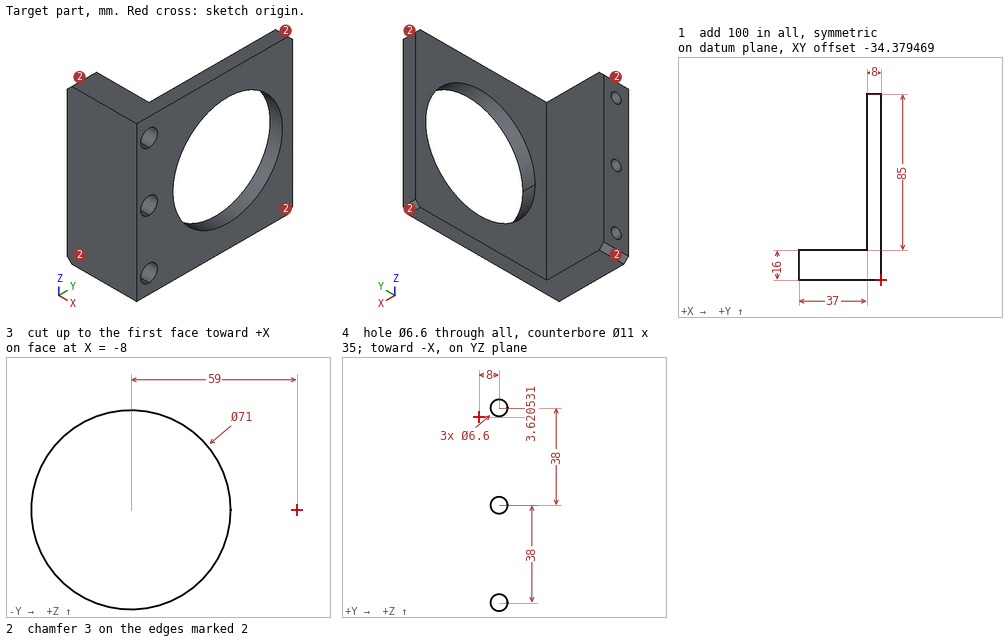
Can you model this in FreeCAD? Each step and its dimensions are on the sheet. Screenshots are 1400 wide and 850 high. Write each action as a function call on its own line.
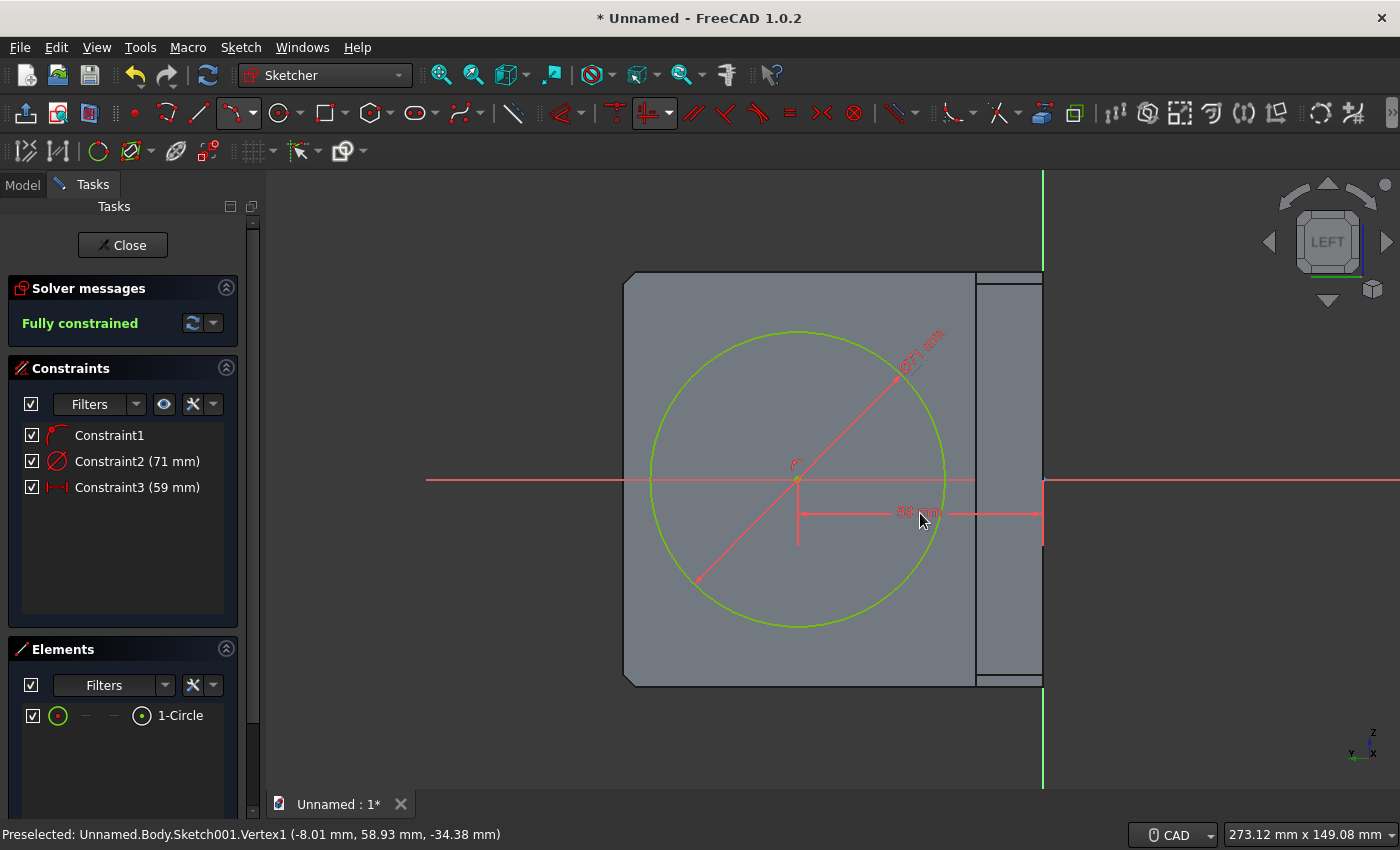
click(123, 245)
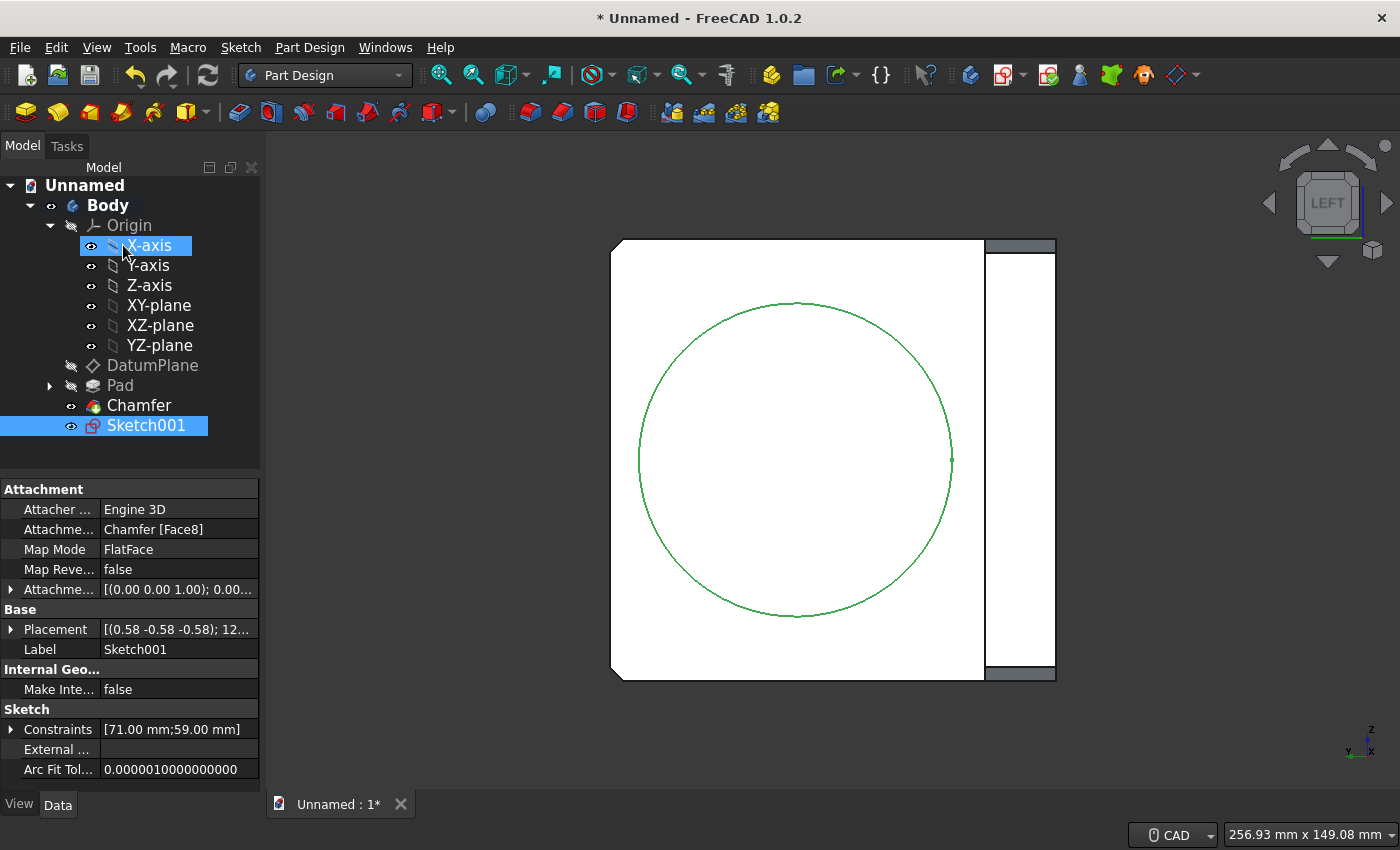
click(240, 112)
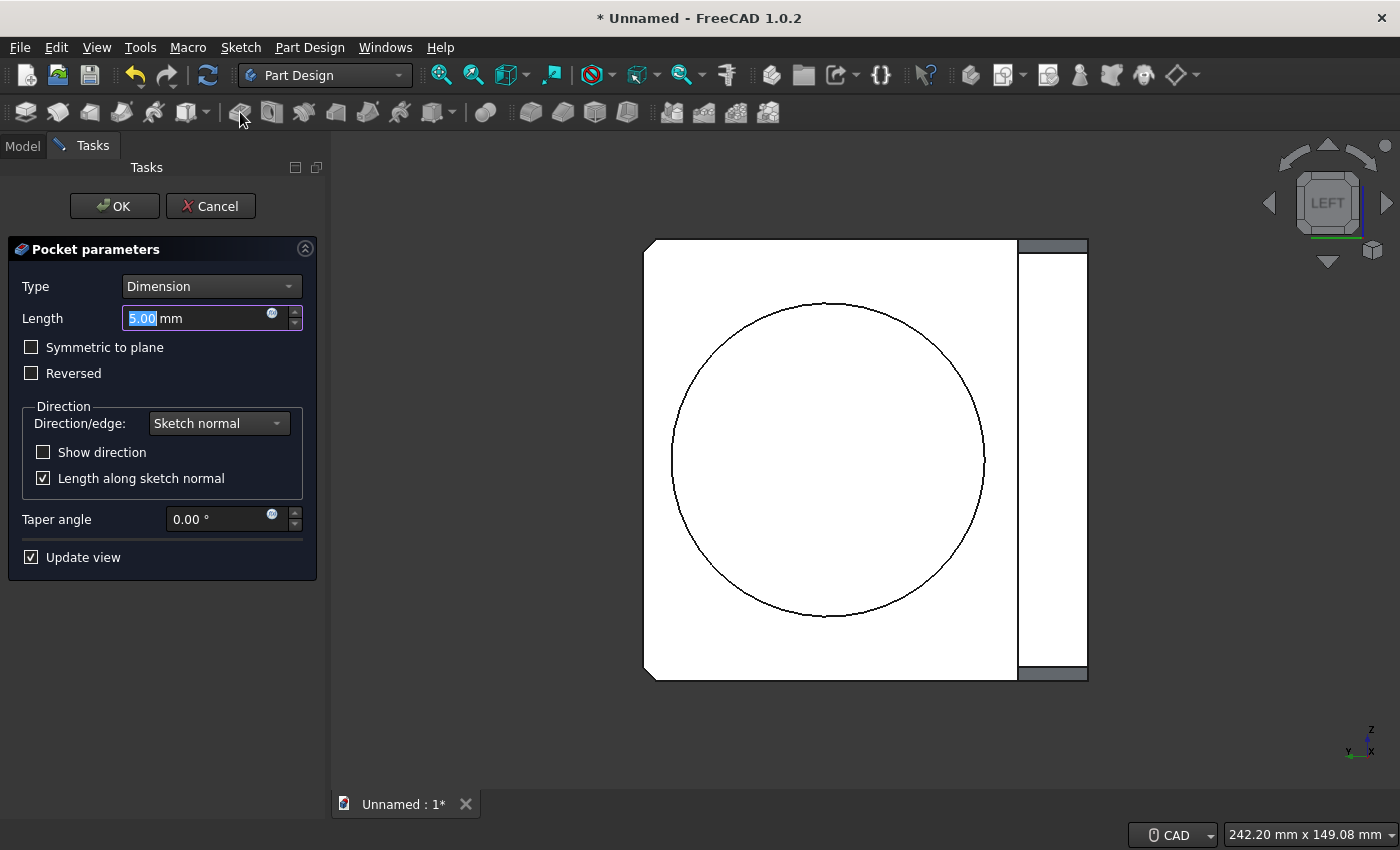
click(212, 286)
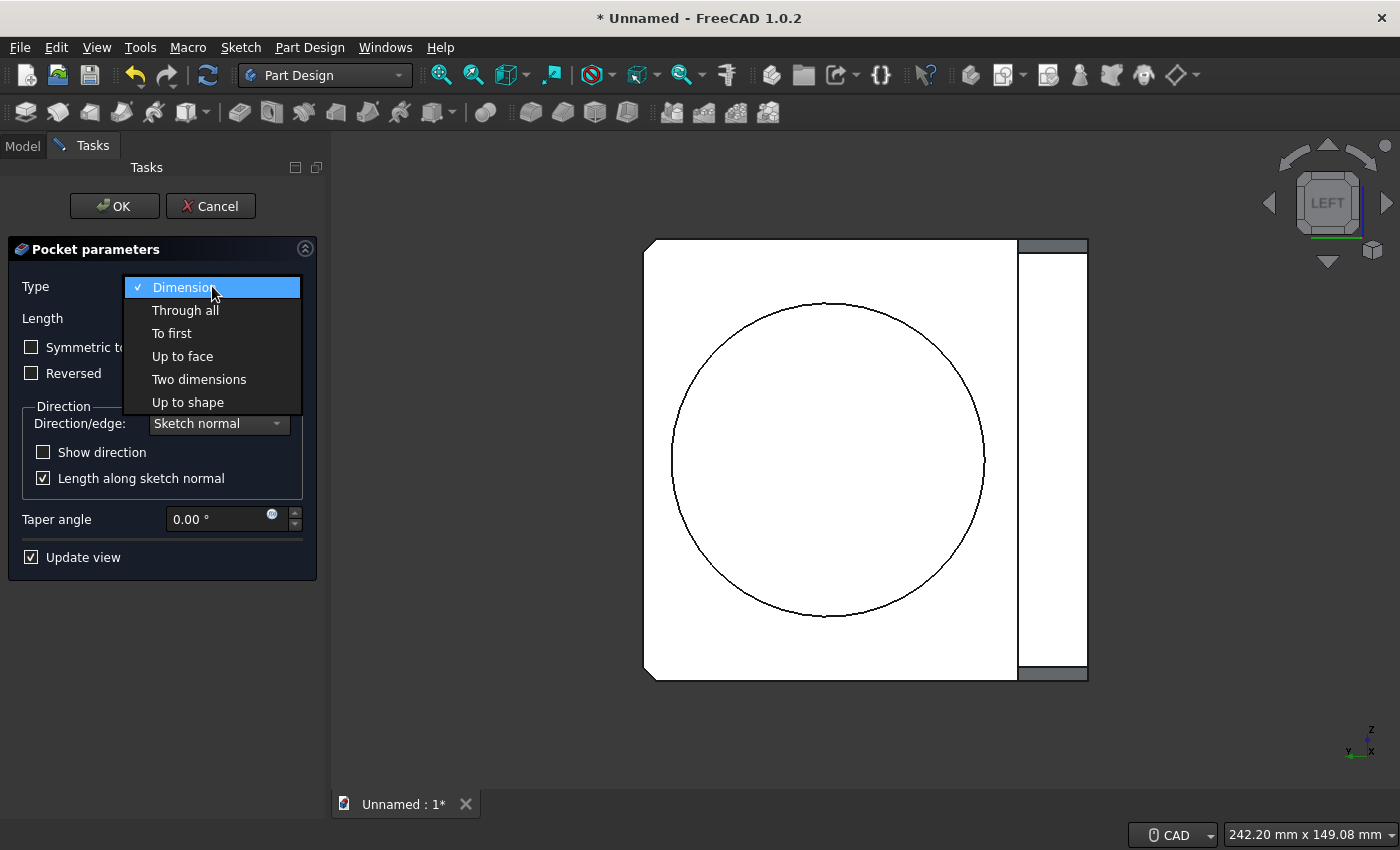
click(212, 334)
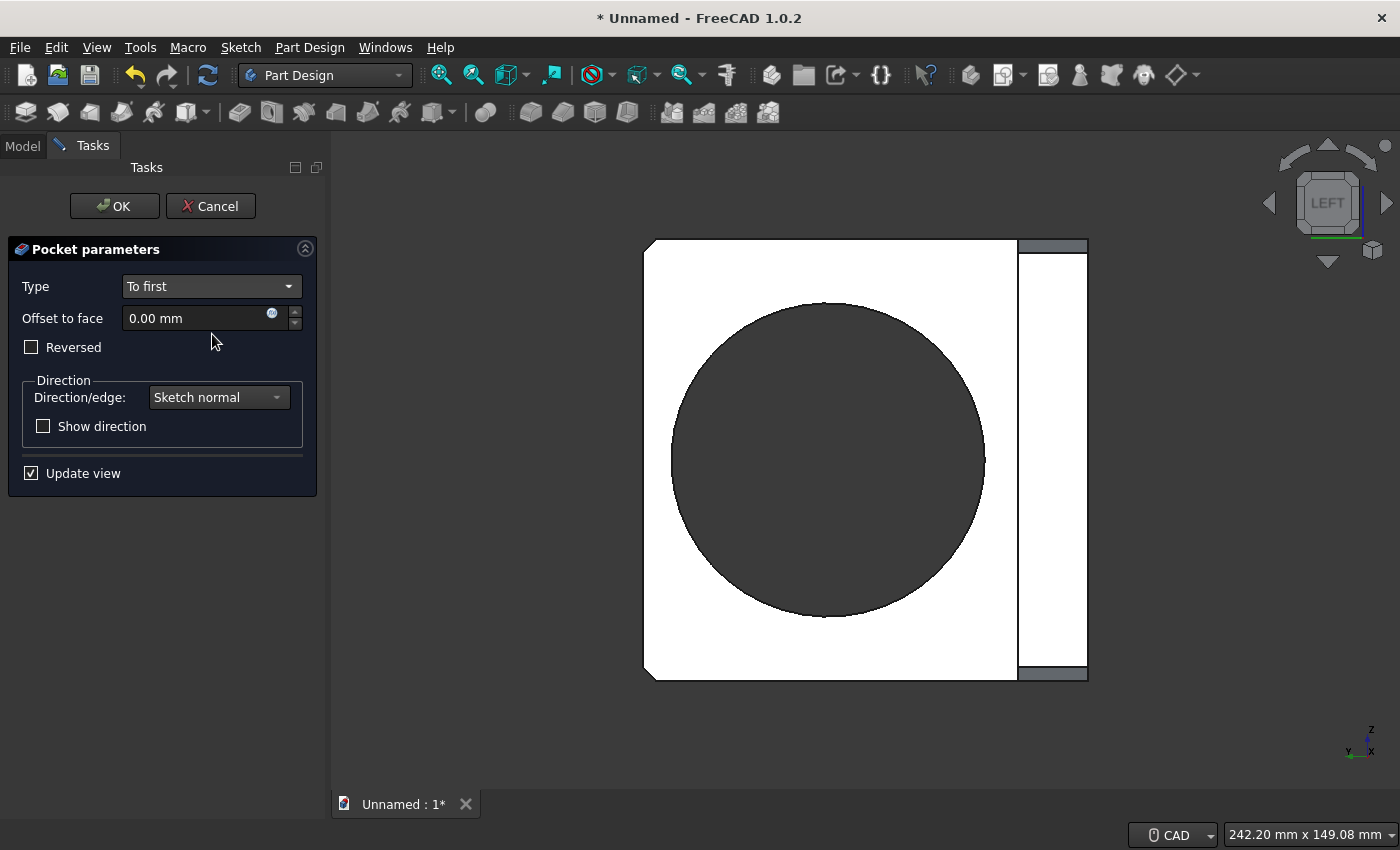
click(115, 206)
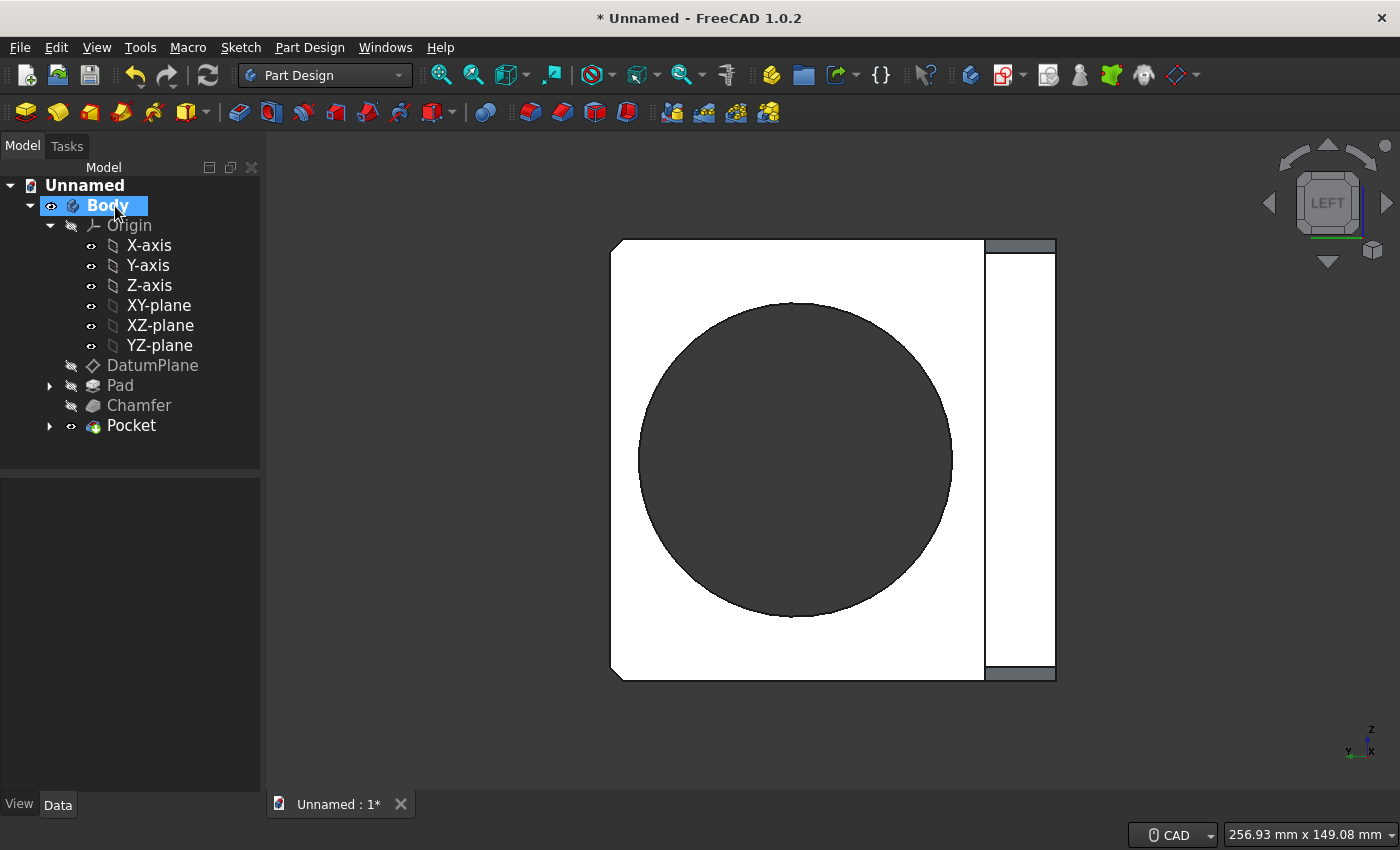
click(1004, 76)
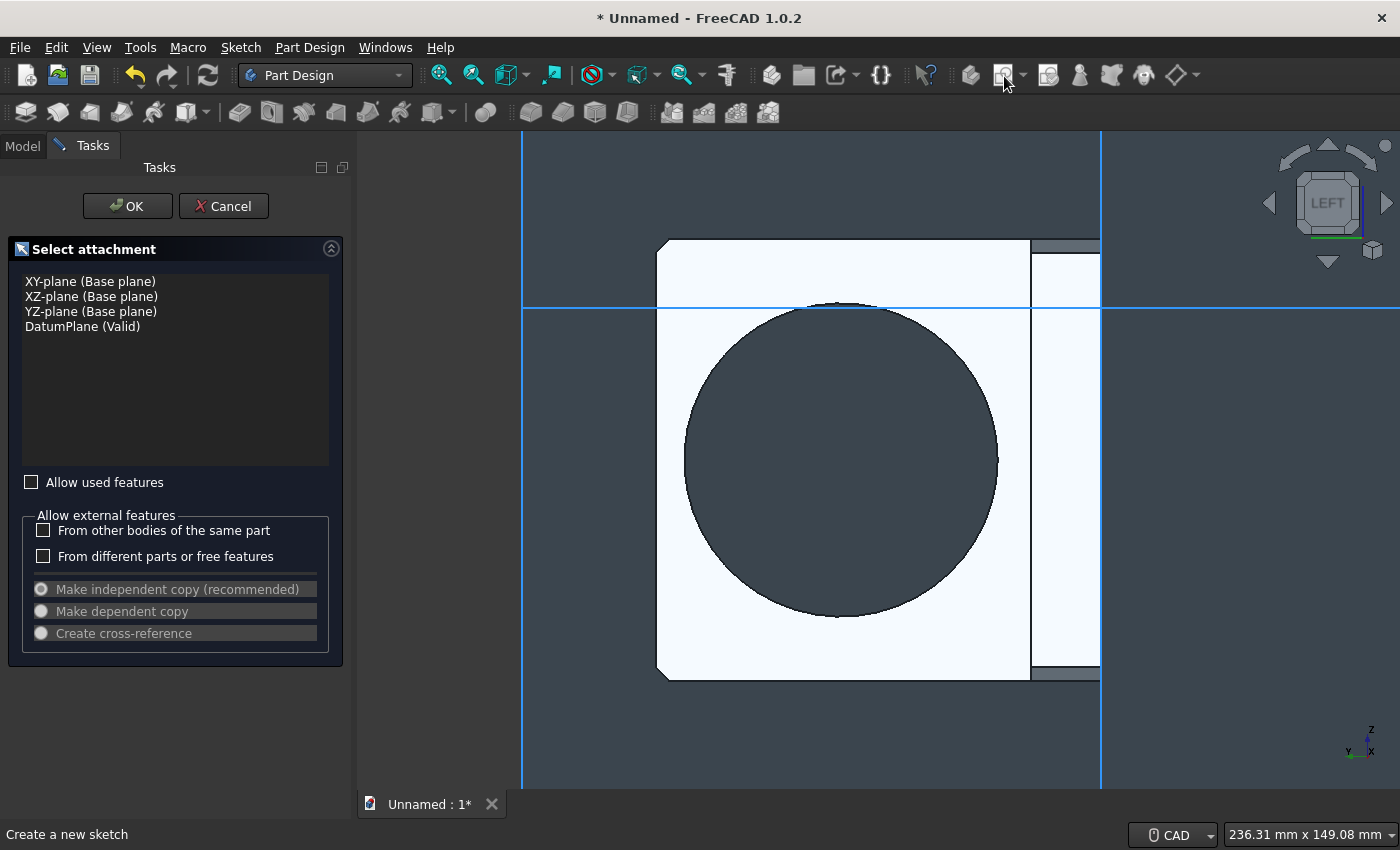
click(82, 312)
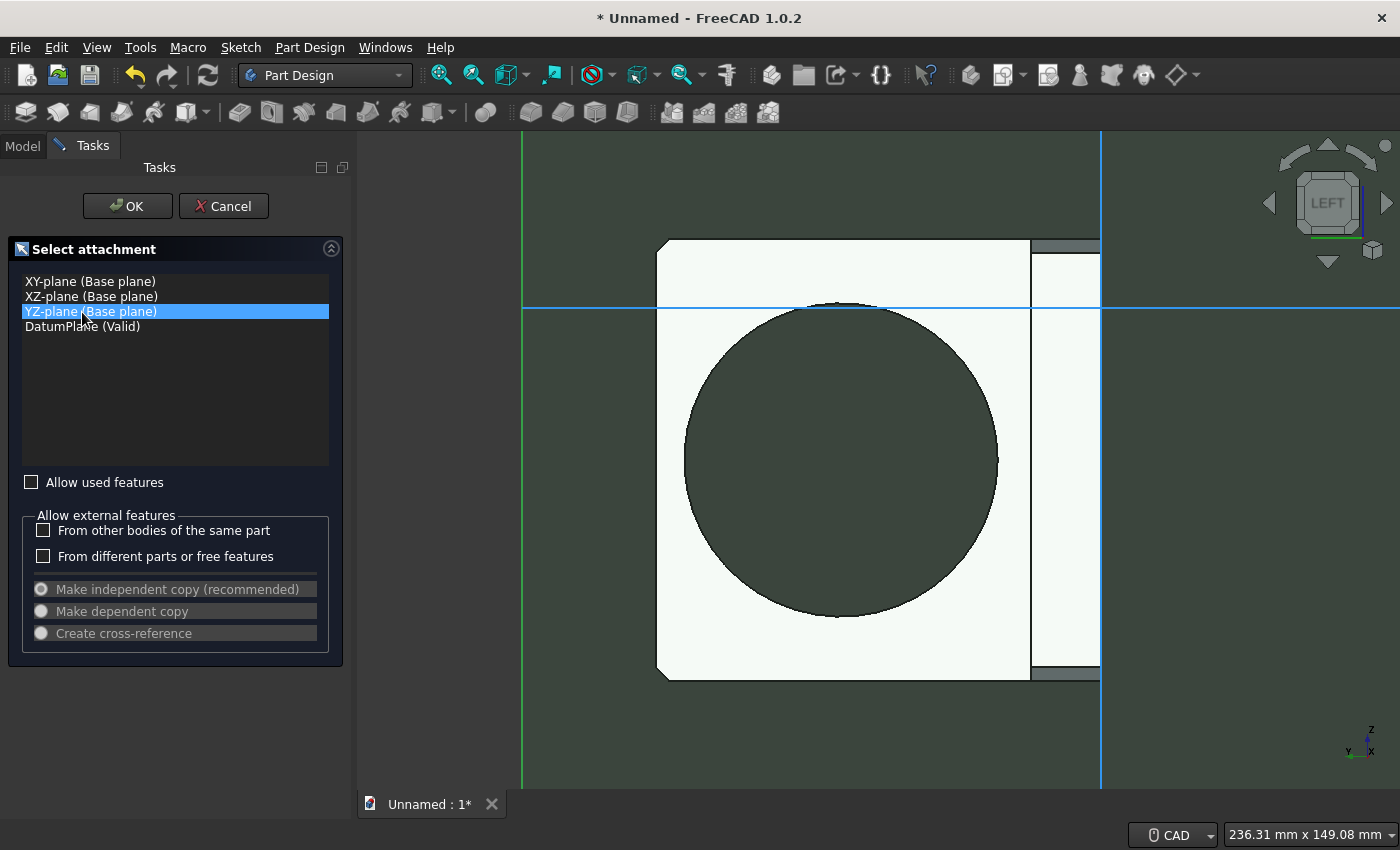
click(128, 206)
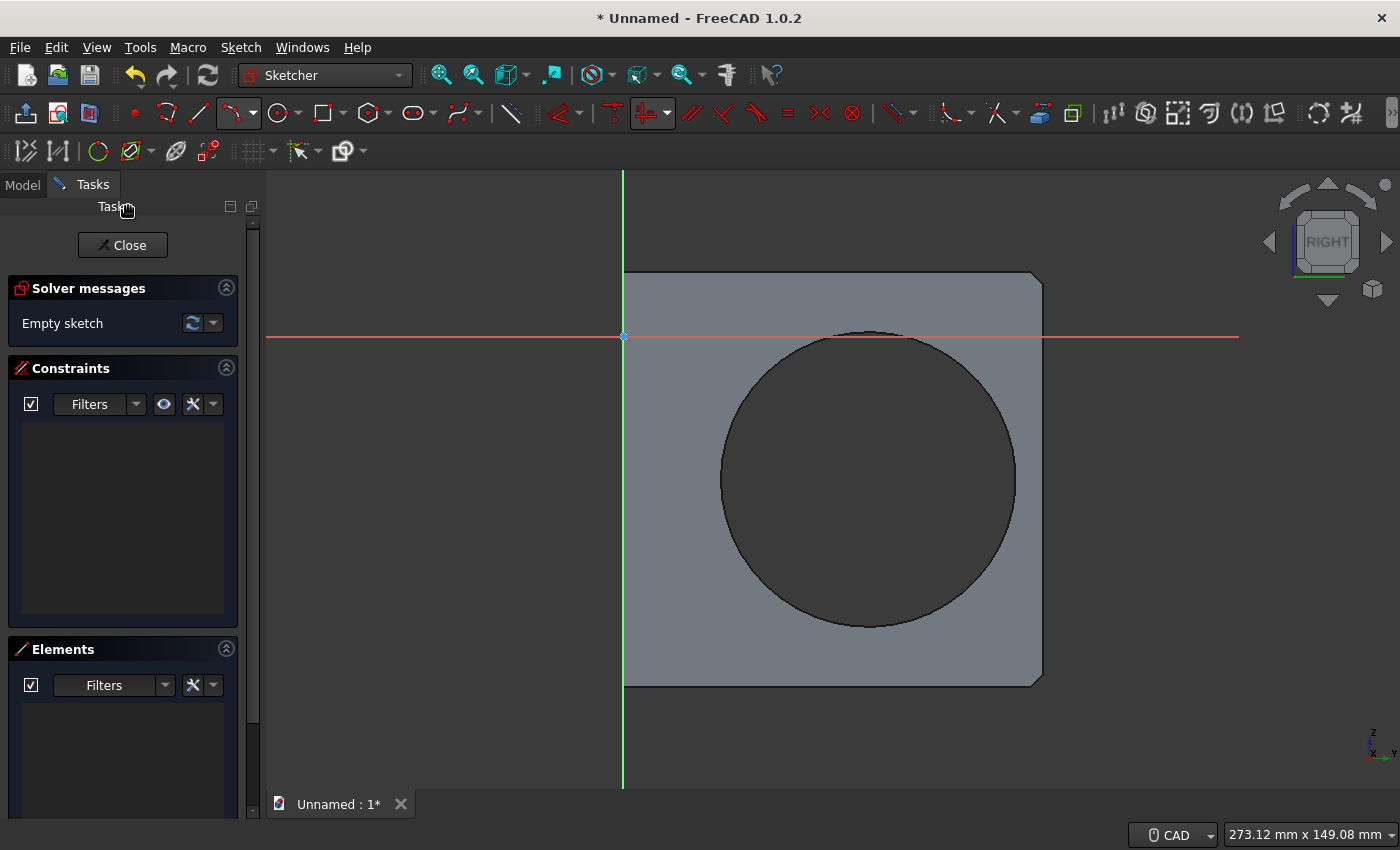
click(278, 114)